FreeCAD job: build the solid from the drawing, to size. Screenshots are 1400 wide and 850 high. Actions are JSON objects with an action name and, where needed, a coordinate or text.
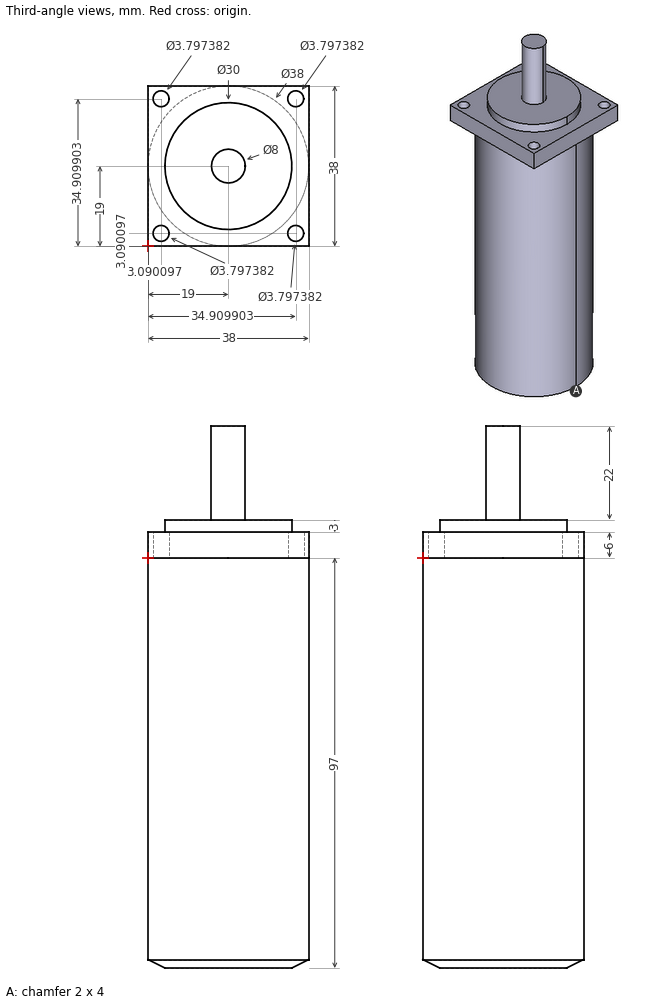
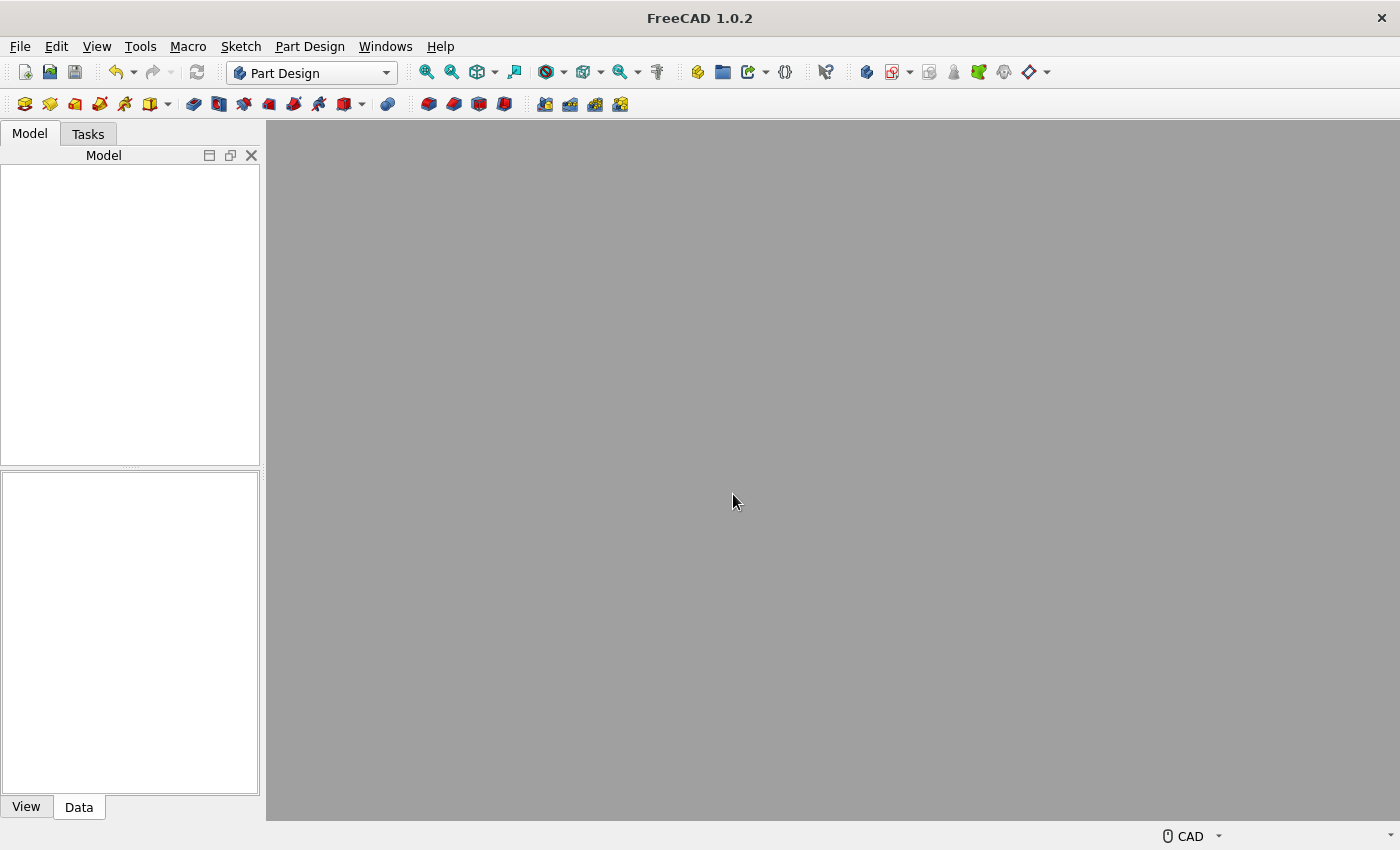
{"action": "key", "text": "ctrl+n"}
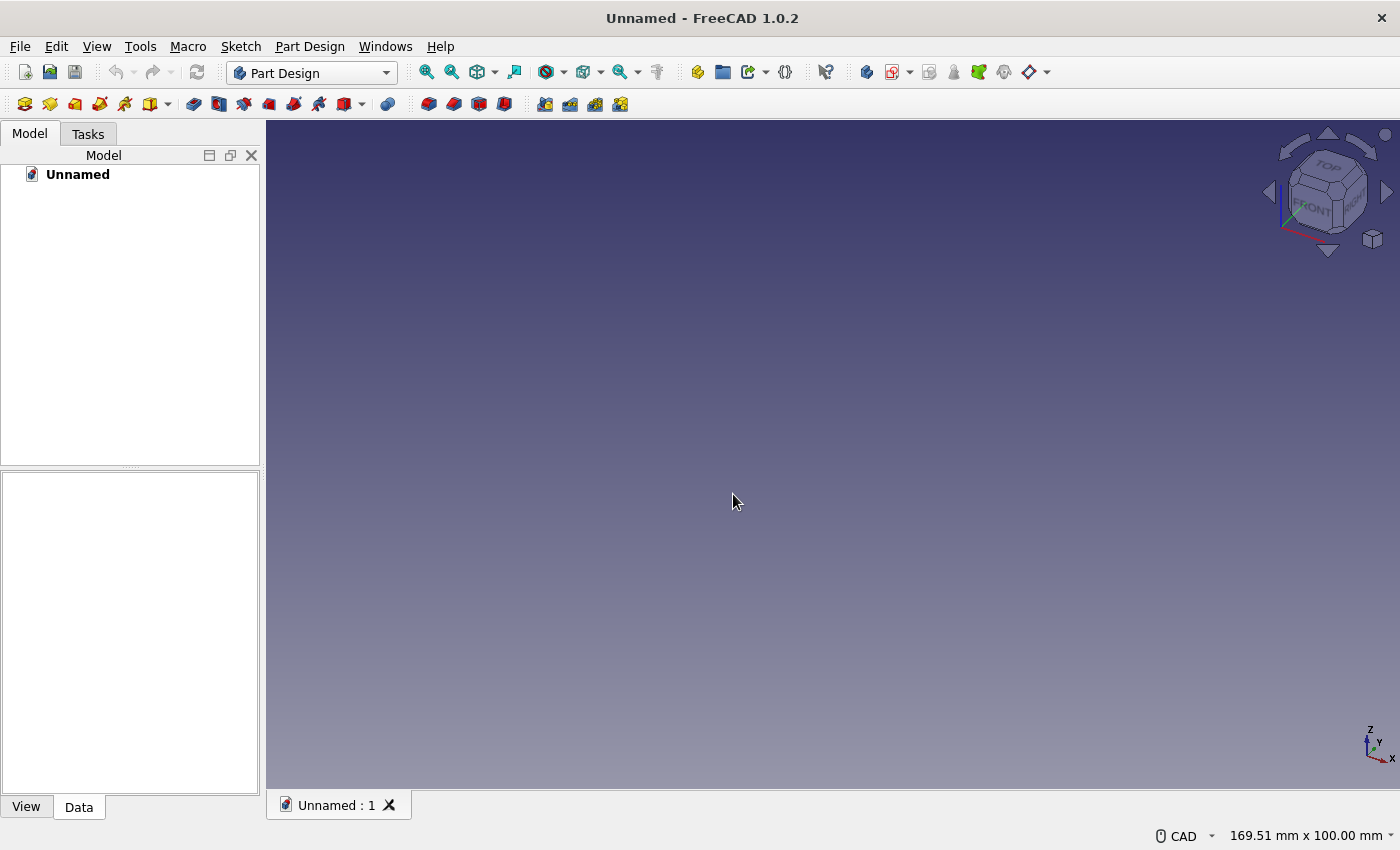
{"action": "left_click", "coordinate": [892, 72]}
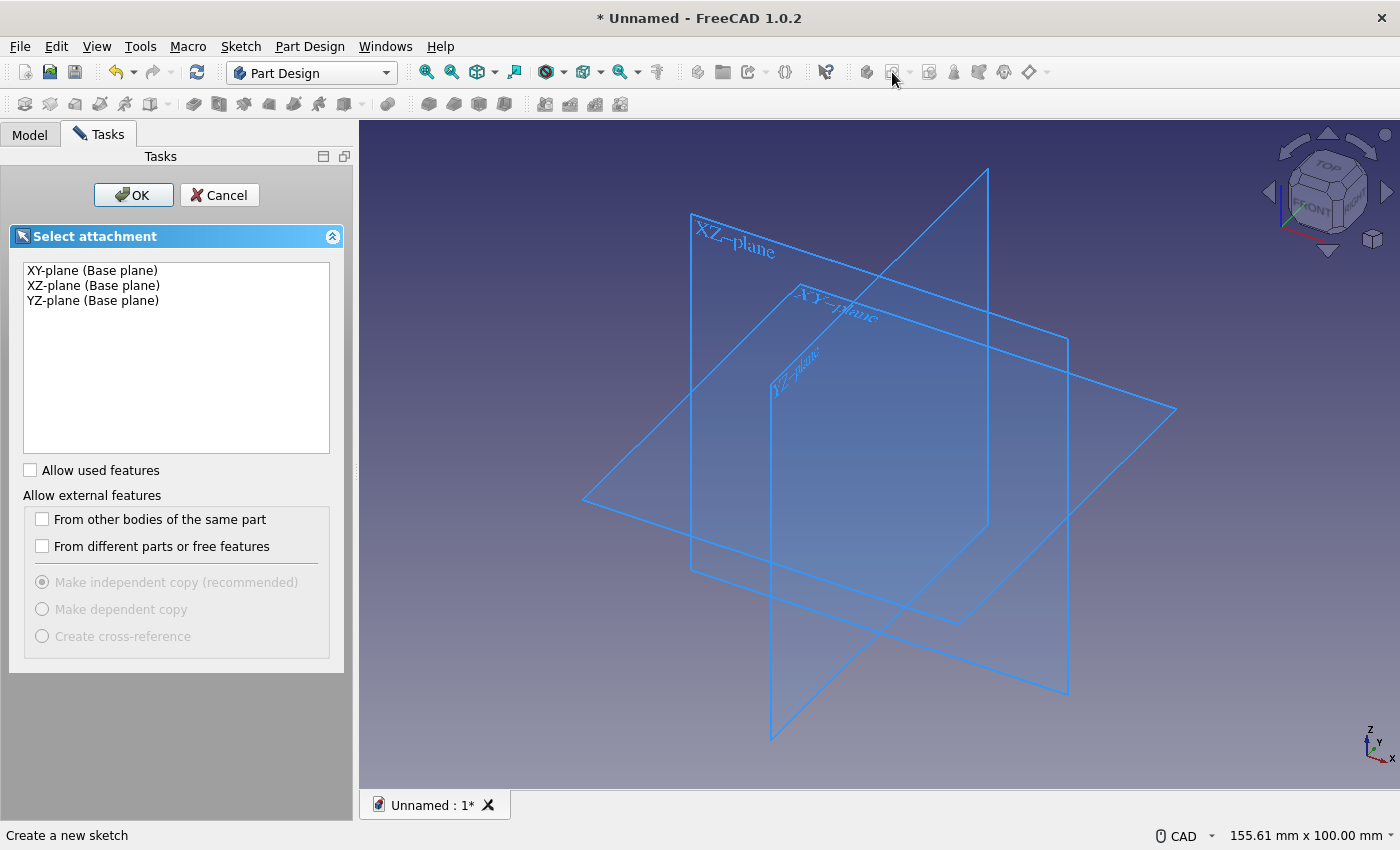
{"action": "left_click", "coordinate": [84, 270]}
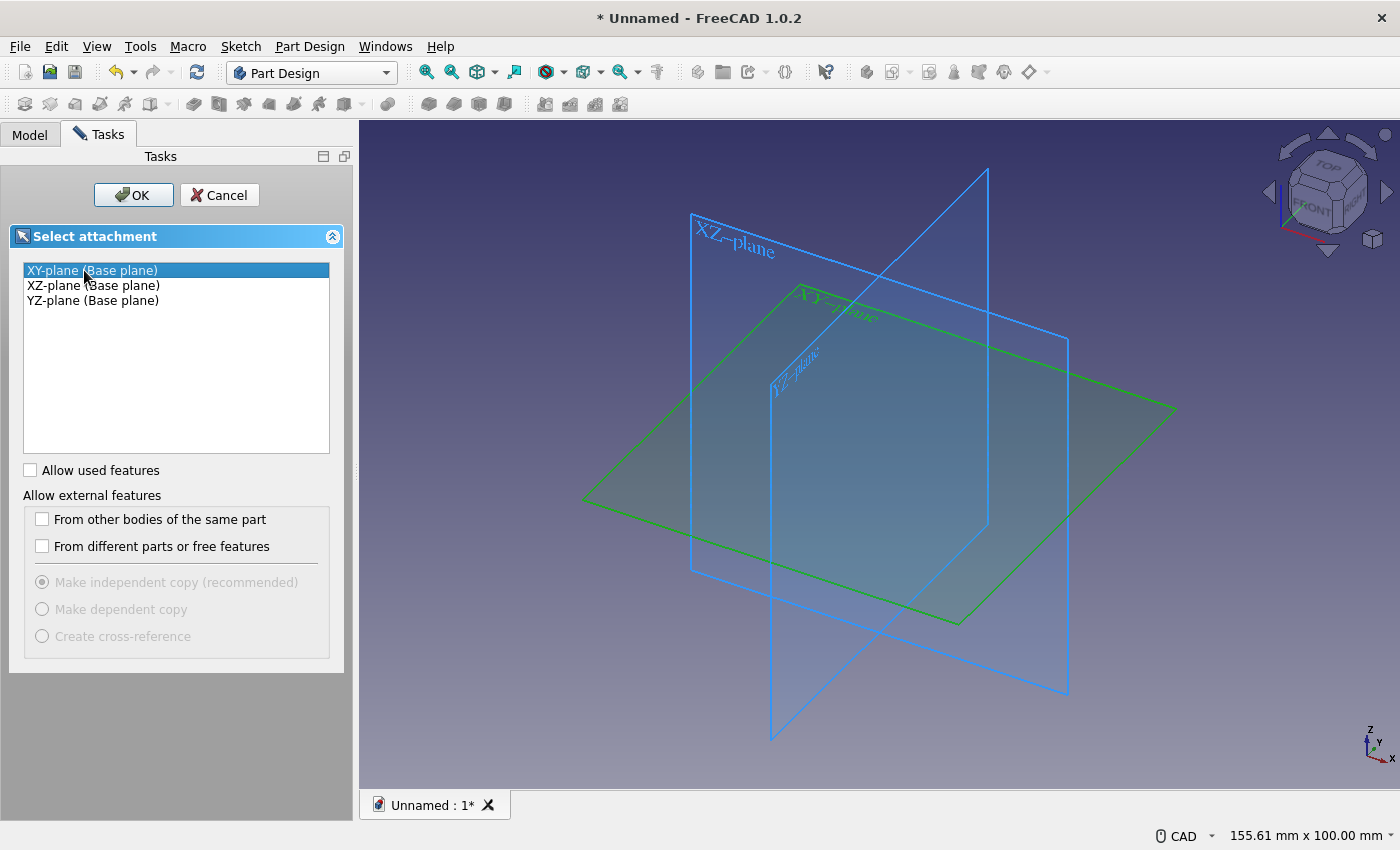
{"action": "left_click", "coordinate": [134, 195]}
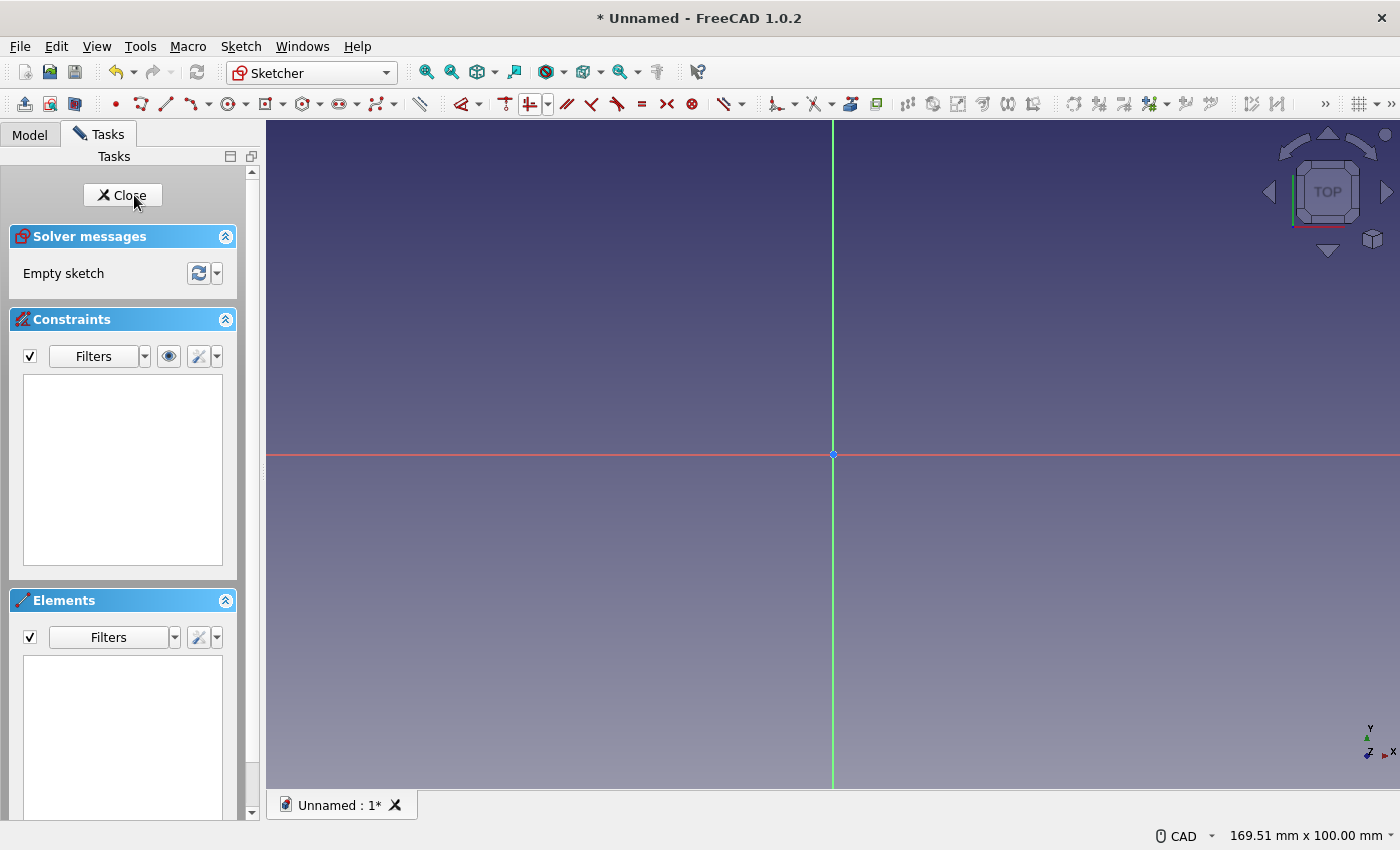
{"action": "scroll", "coordinate": [1198, 173], "scroll_direction": "up", "scroll_amount": 3}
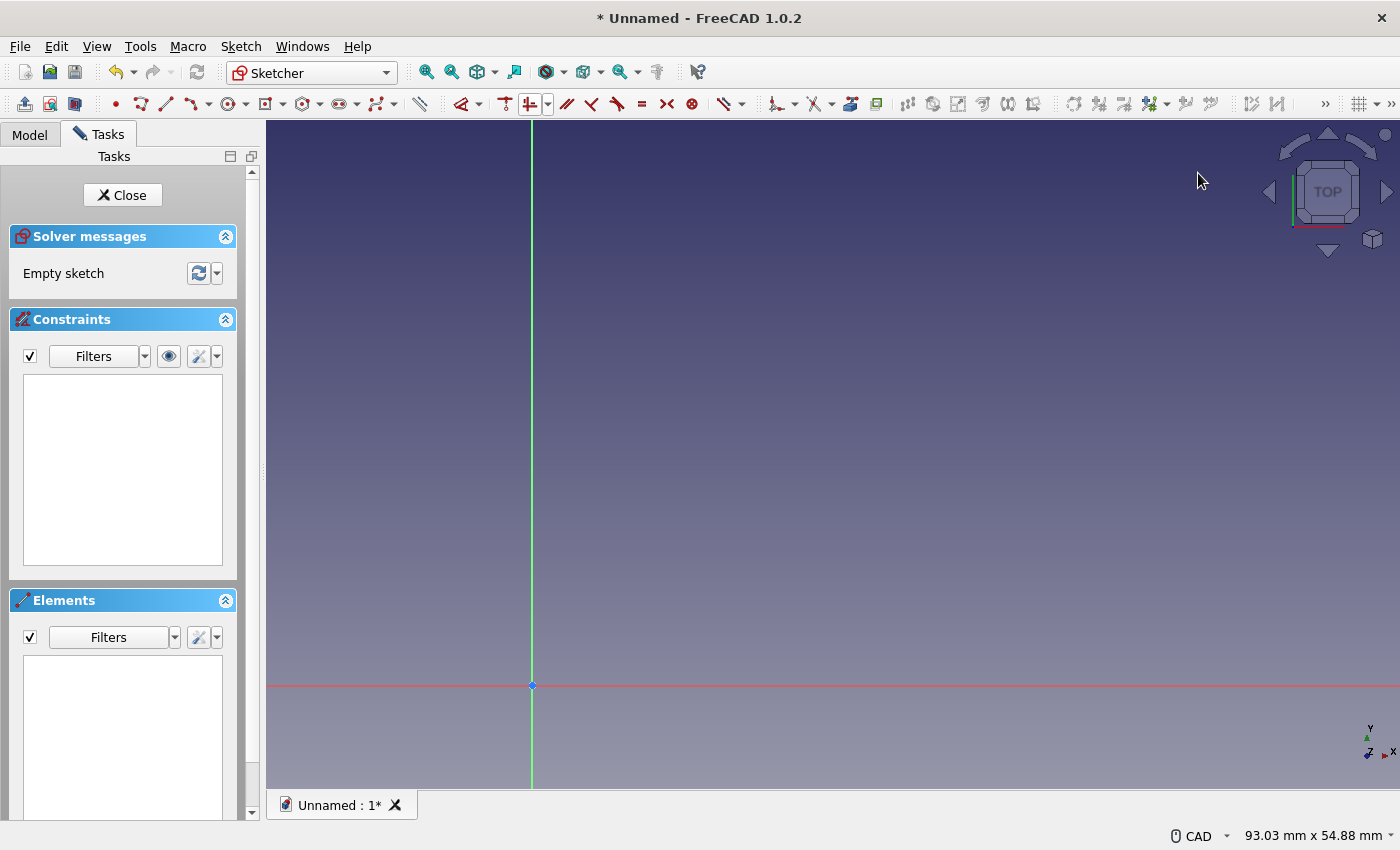
{"action": "key", "text": "g r"}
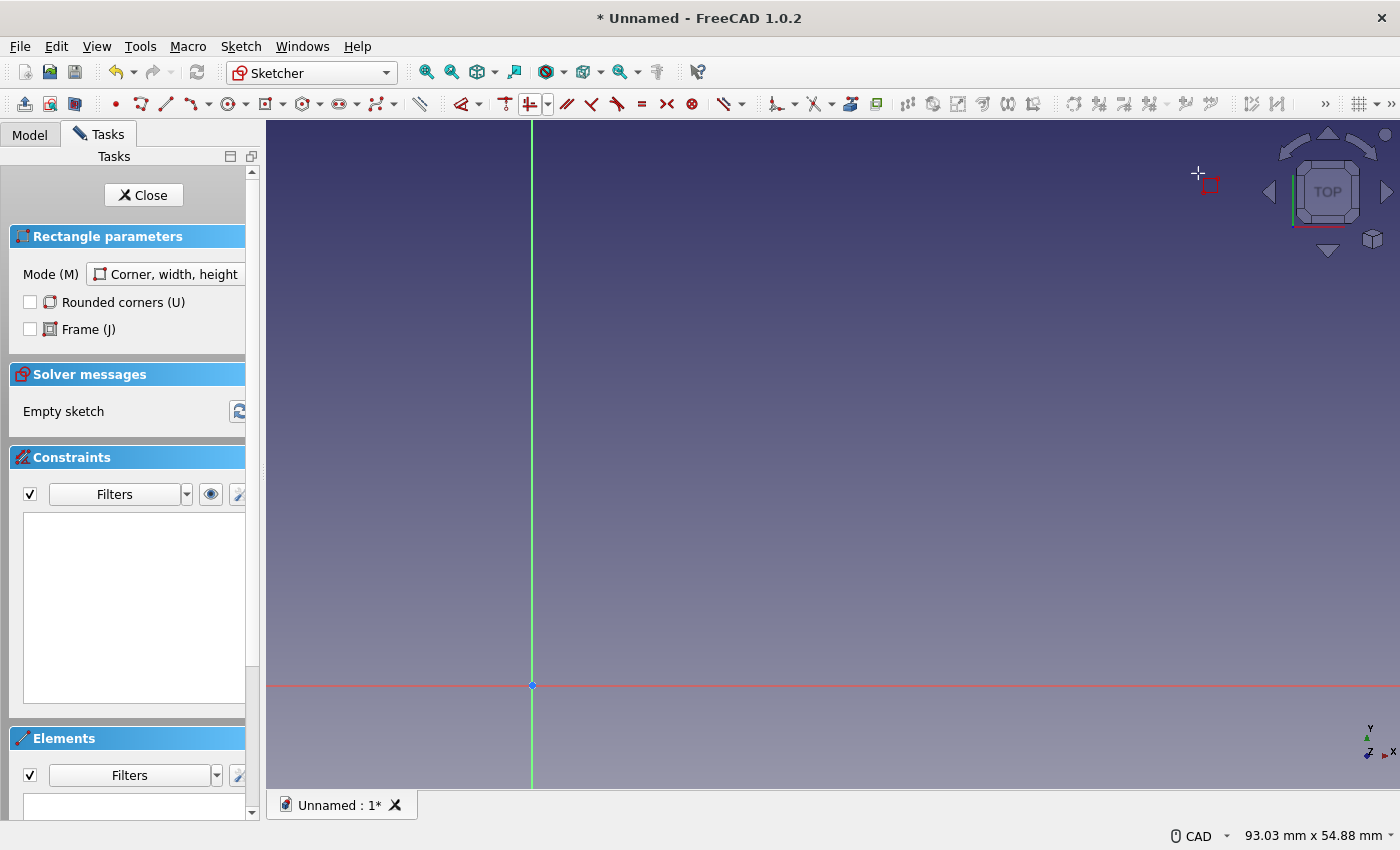
{"action": "left_click", "coordinate": [532, 686]}
{"action": "mouse_move", "coordinate": [995, 223]}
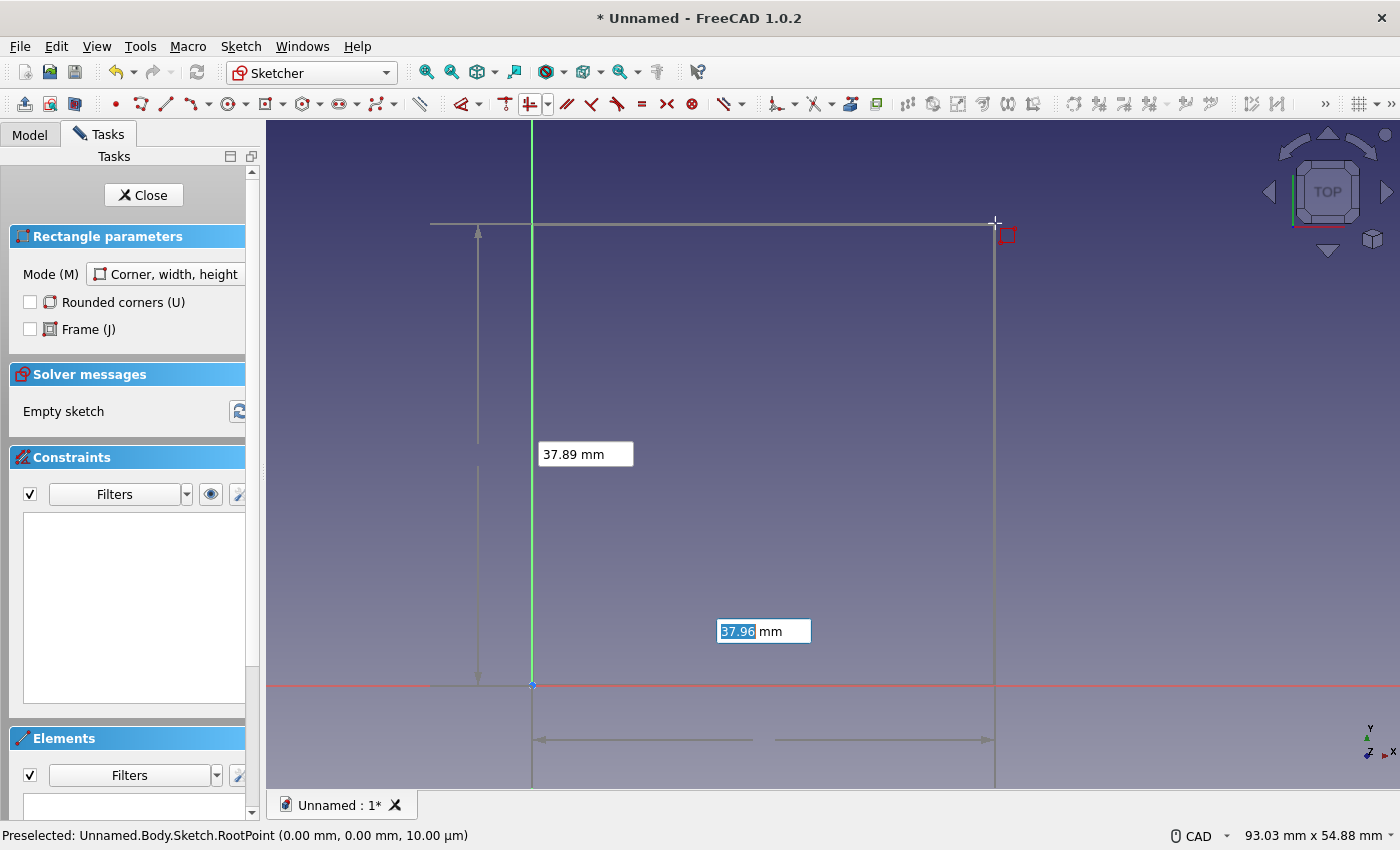
{"action": "type", "text": "38"}
{"action": "key", "text": "Tab"}
{"action": "type", "text": "38"}
{"action": "key", "text": "Return"}
{"action": "key", "text": "Escape"}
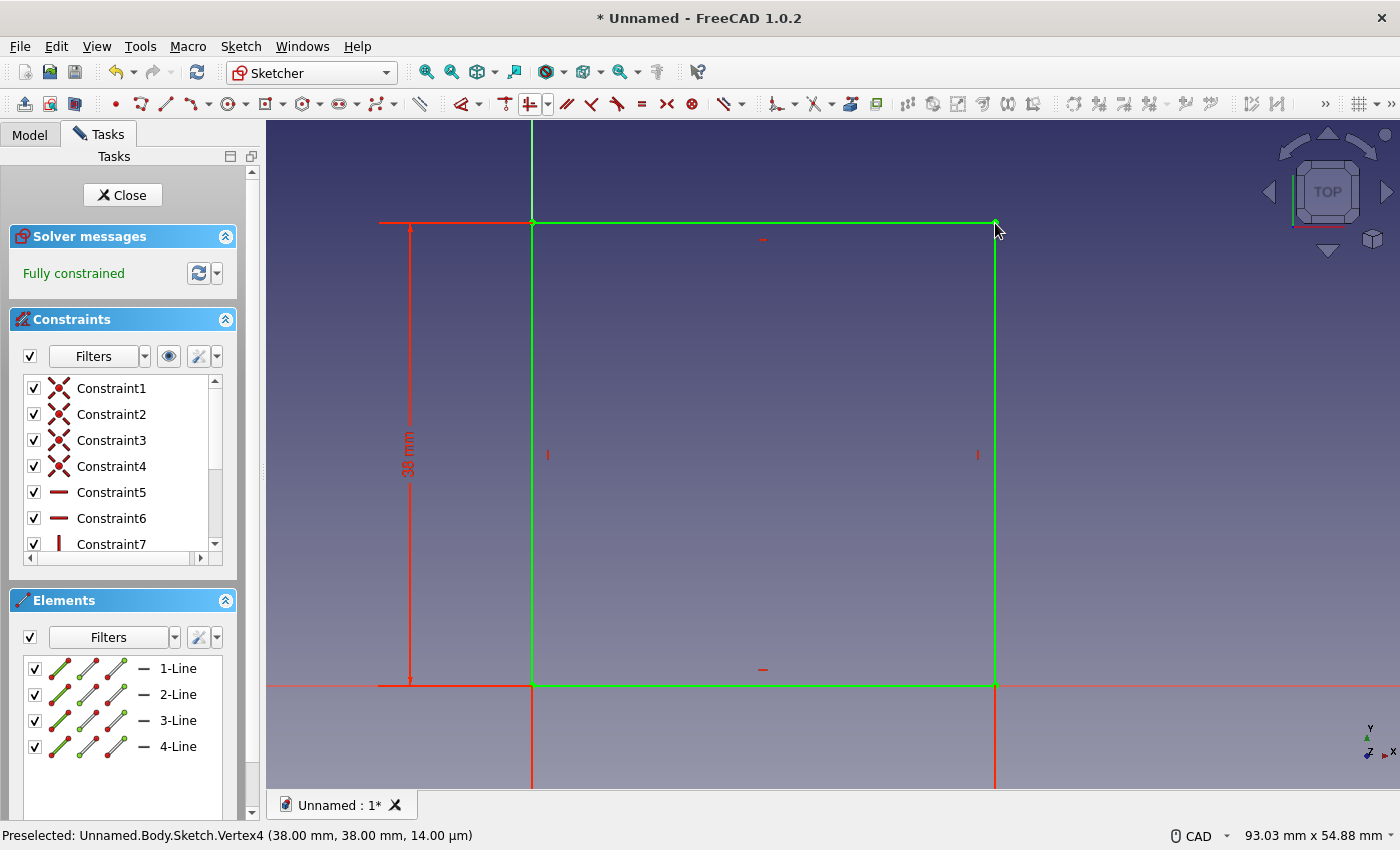
{"action": "left_click", "coordinate": [123, 195]}